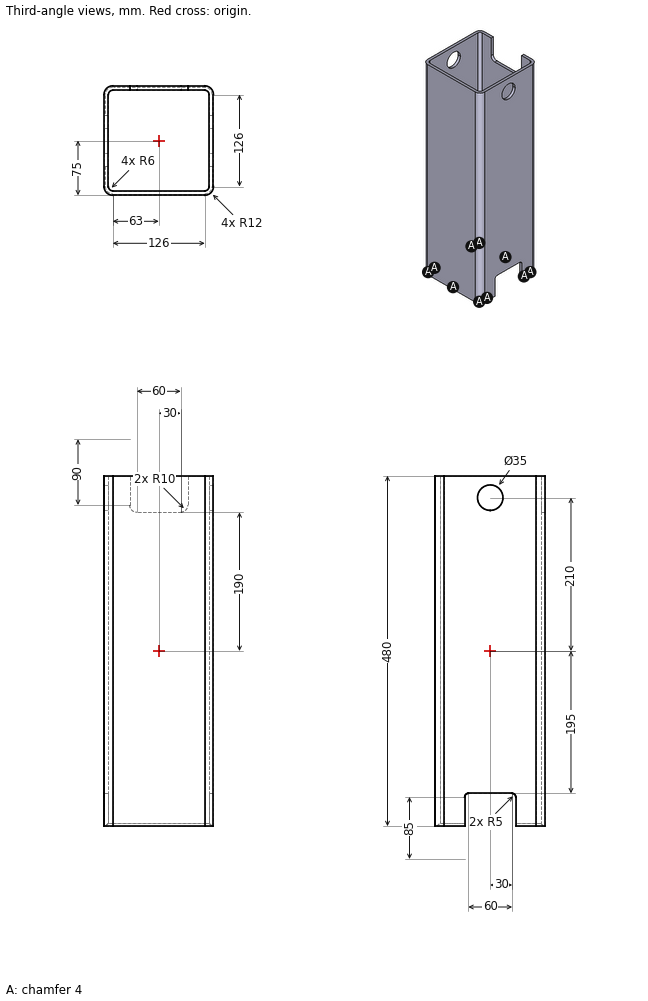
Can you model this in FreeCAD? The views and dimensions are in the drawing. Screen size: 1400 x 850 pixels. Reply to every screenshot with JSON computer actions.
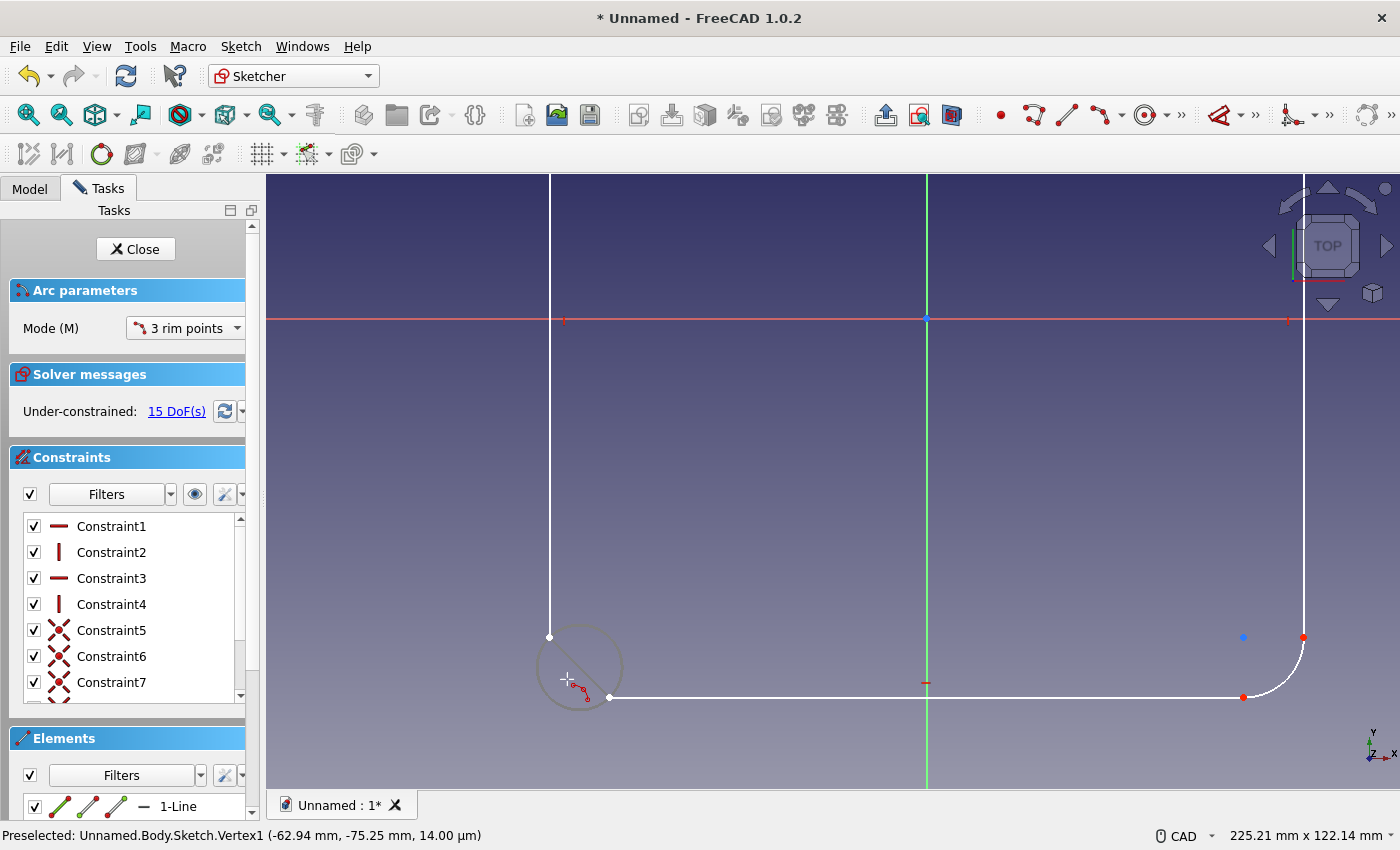
{"action": "left_click", "coordinate": [567, 679]}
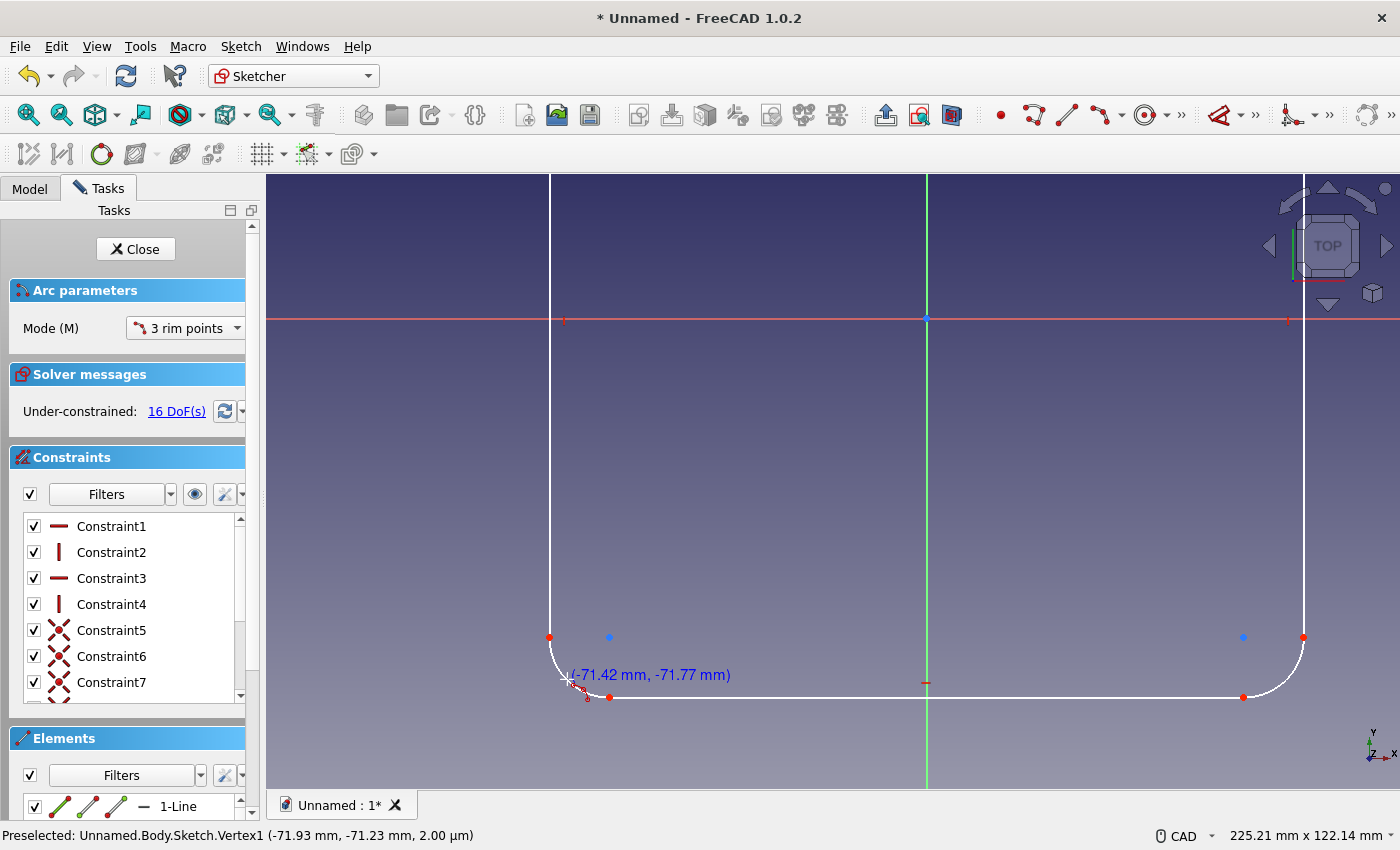
{"action": "key", "text": "g l"}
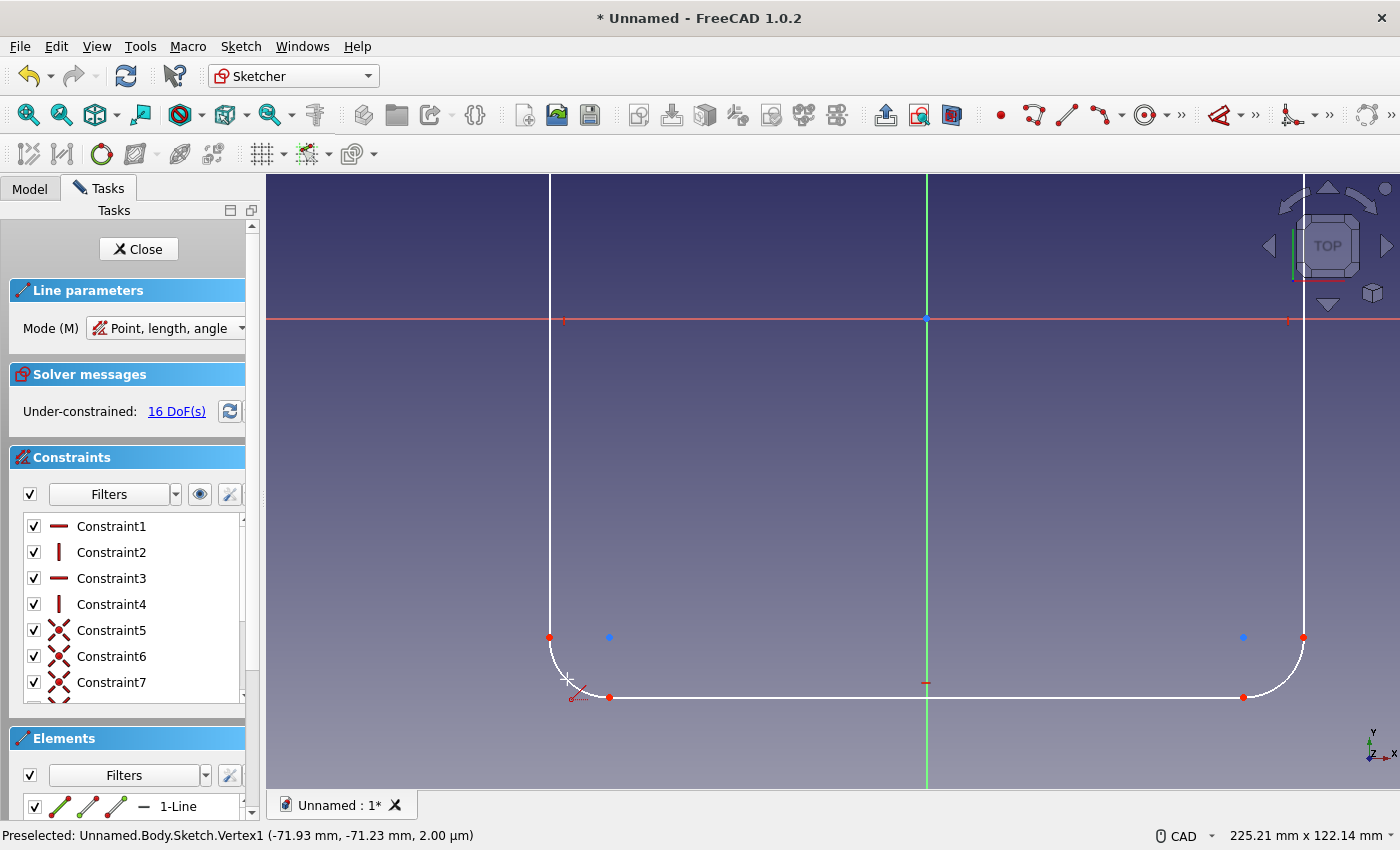
{"action": "scroll", "coordinate": [567, 680], "scroll_direction": "down", "scroll_amount": 3}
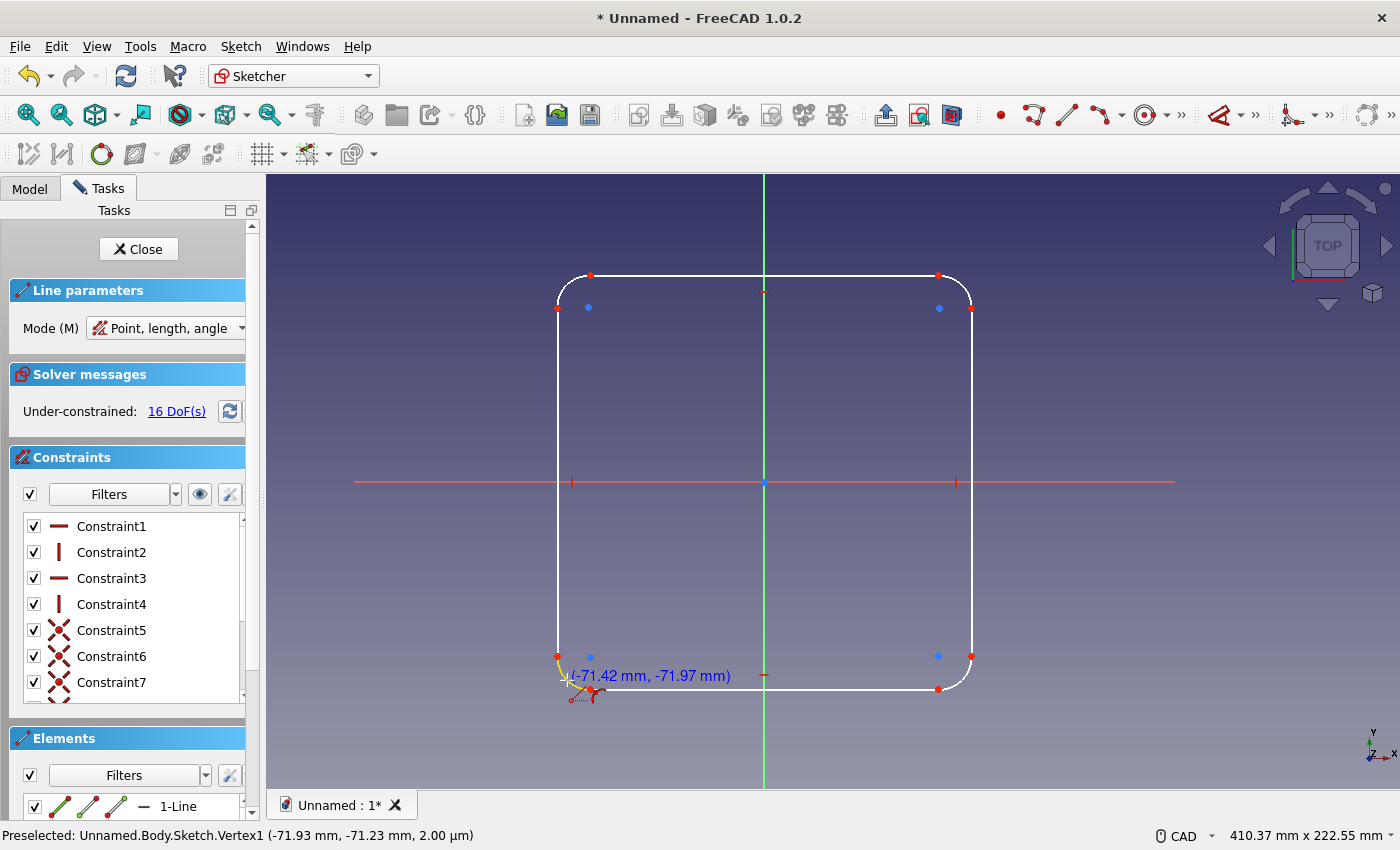
{"action": "left_click", "coordinate": [939, 673]}
{"action": "left_click", "coordinate": [590, 673]}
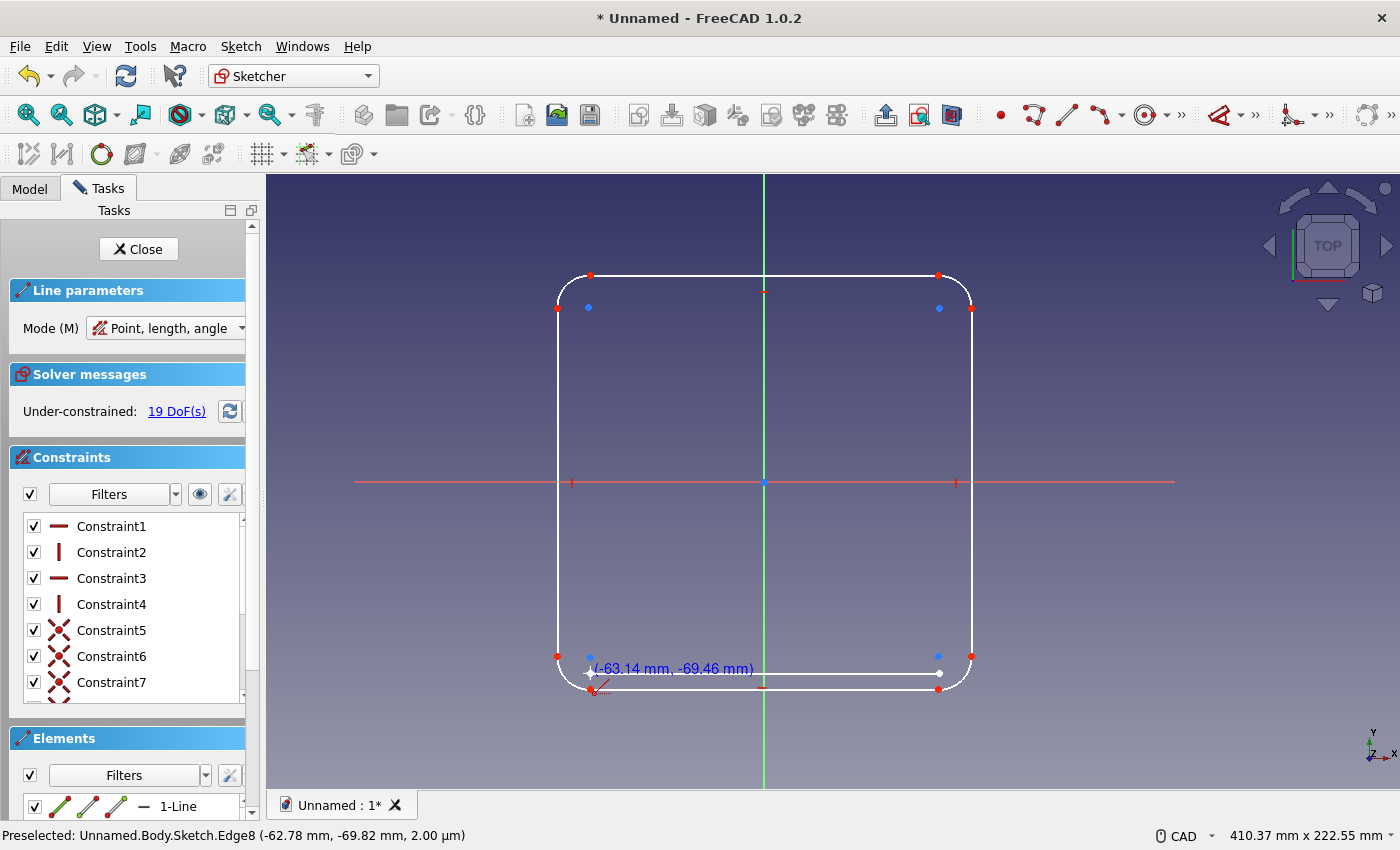
{"action": "left_click", "coordinate": [574, 656]}
{"action": "left_click", "coordinate": [574, 308]}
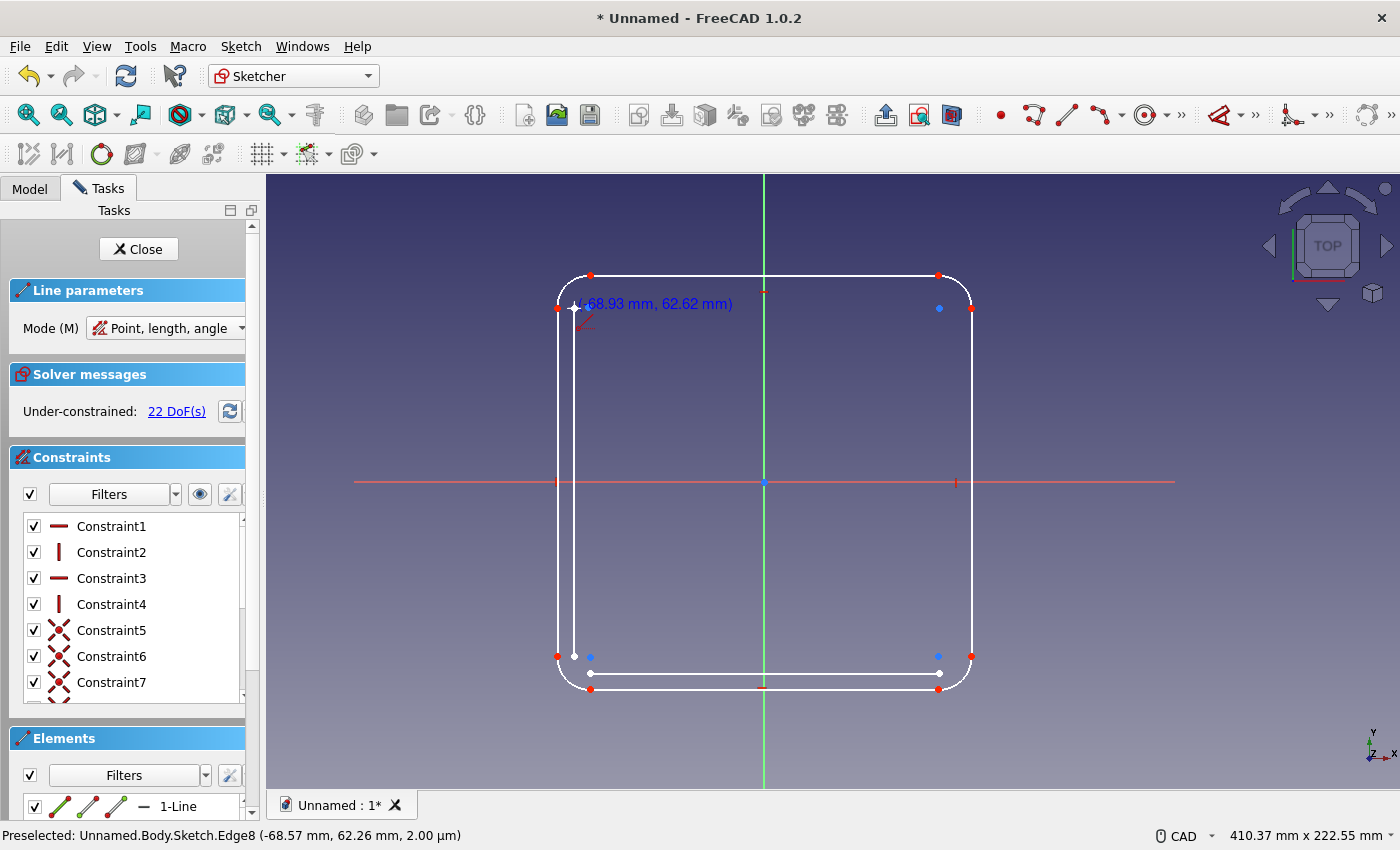
{"action": "left_click", "coordinate": [590, 291]}
{"action": "left_click", "coordinate": [939, 291]}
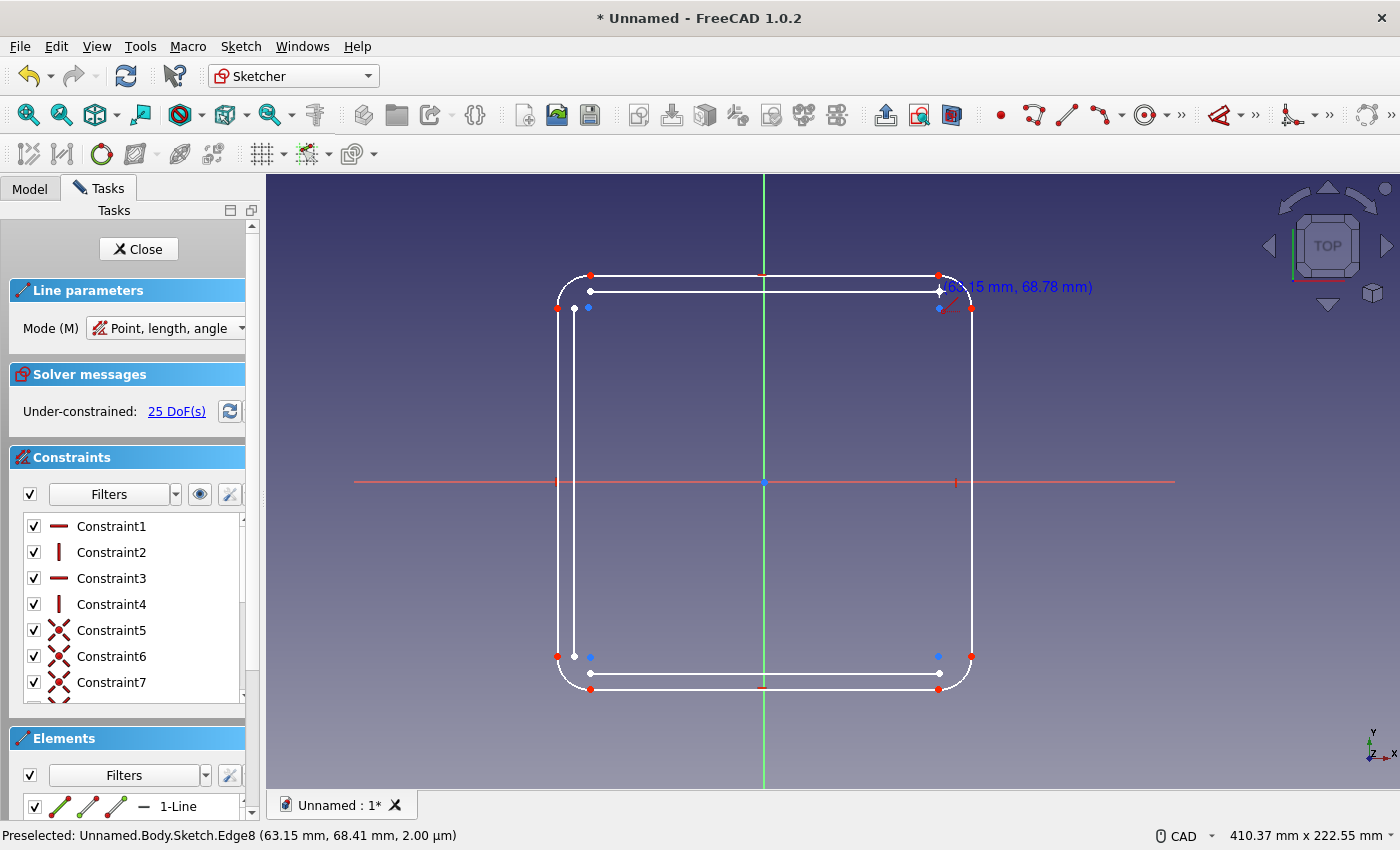
{"action": "left_click", "coordinate": [955, 308]}
{"action": "left_click", "coordinate": [955, 656]}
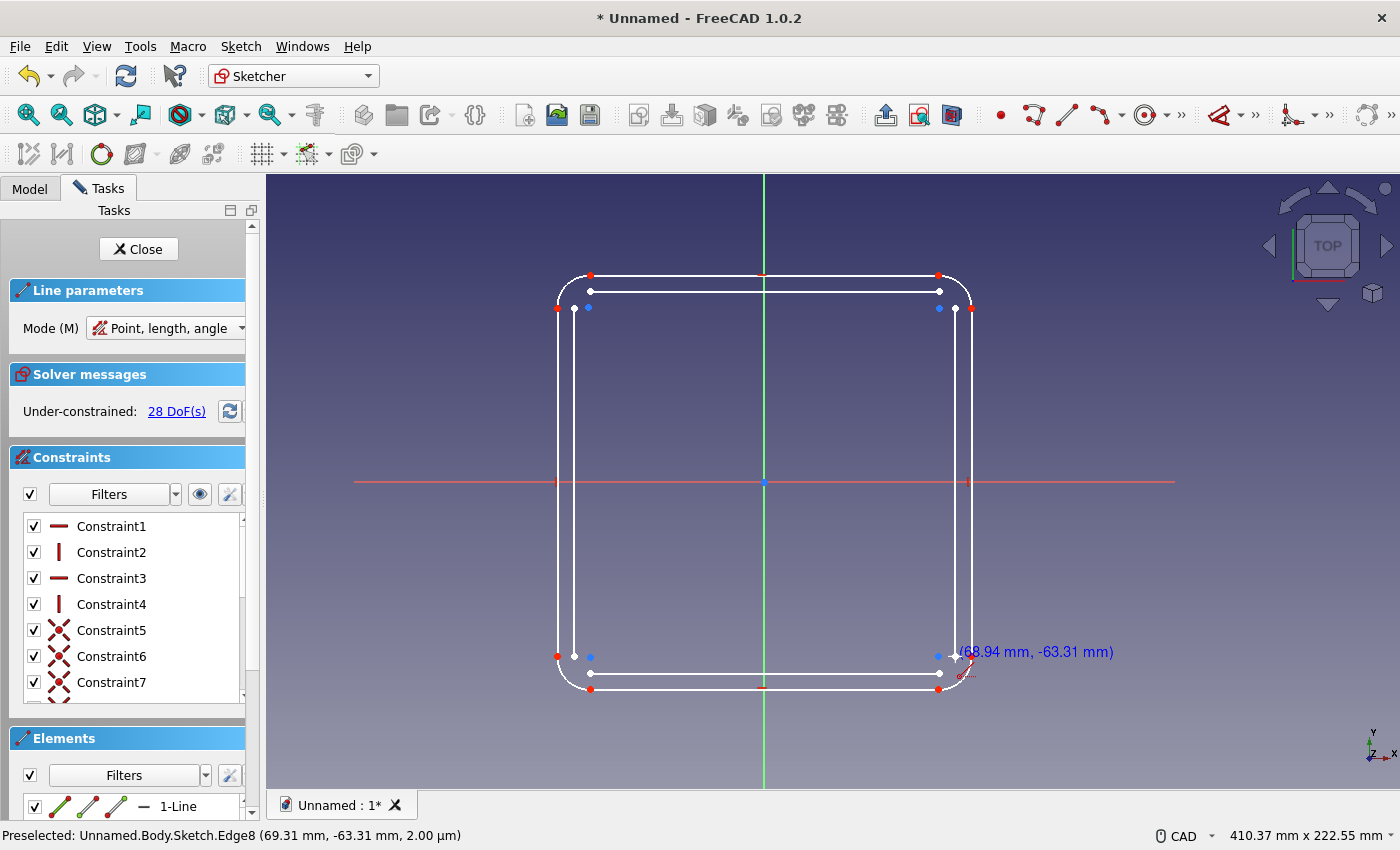
{"action": "left_click", "coordinate": [1100, 116]}